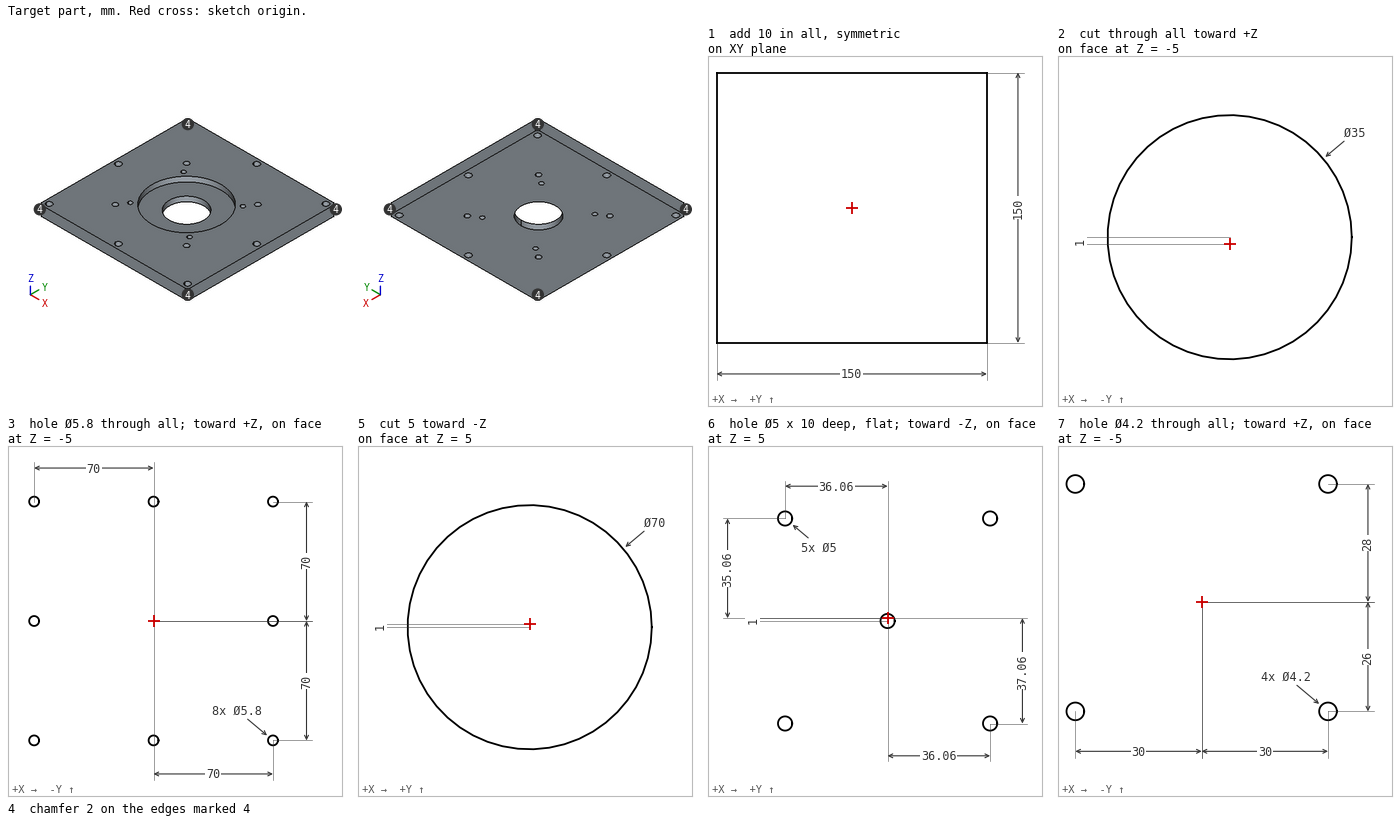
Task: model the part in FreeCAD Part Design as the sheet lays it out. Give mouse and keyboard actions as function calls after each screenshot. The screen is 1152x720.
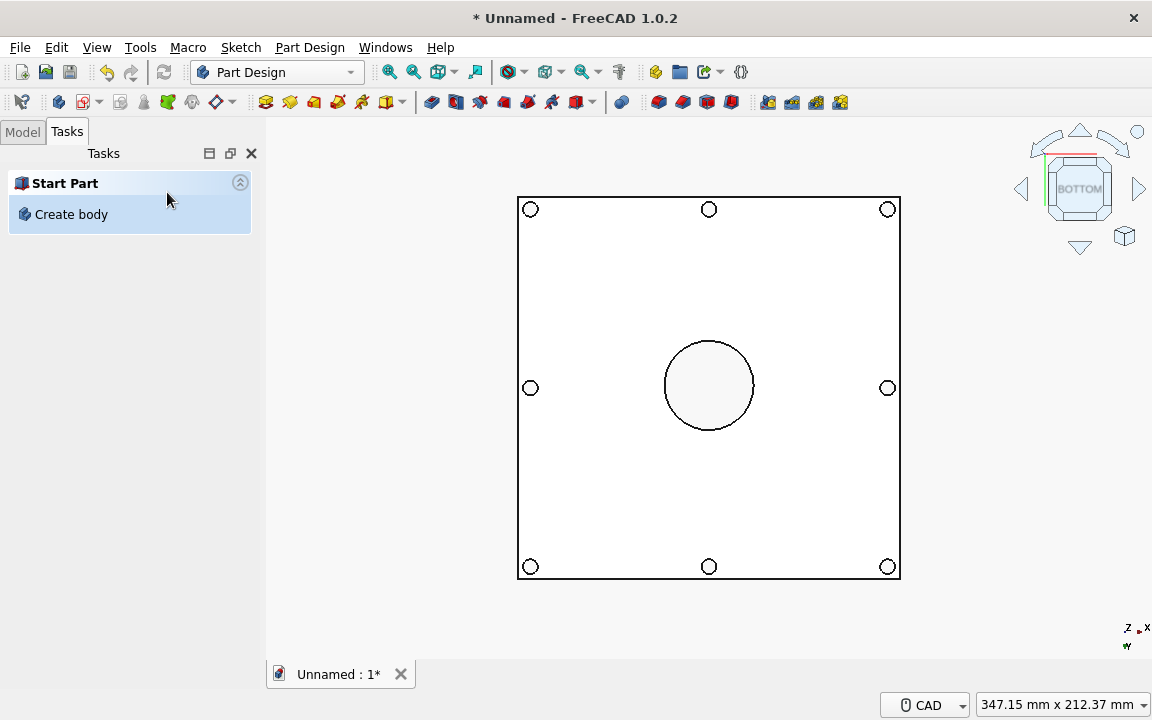
key(0)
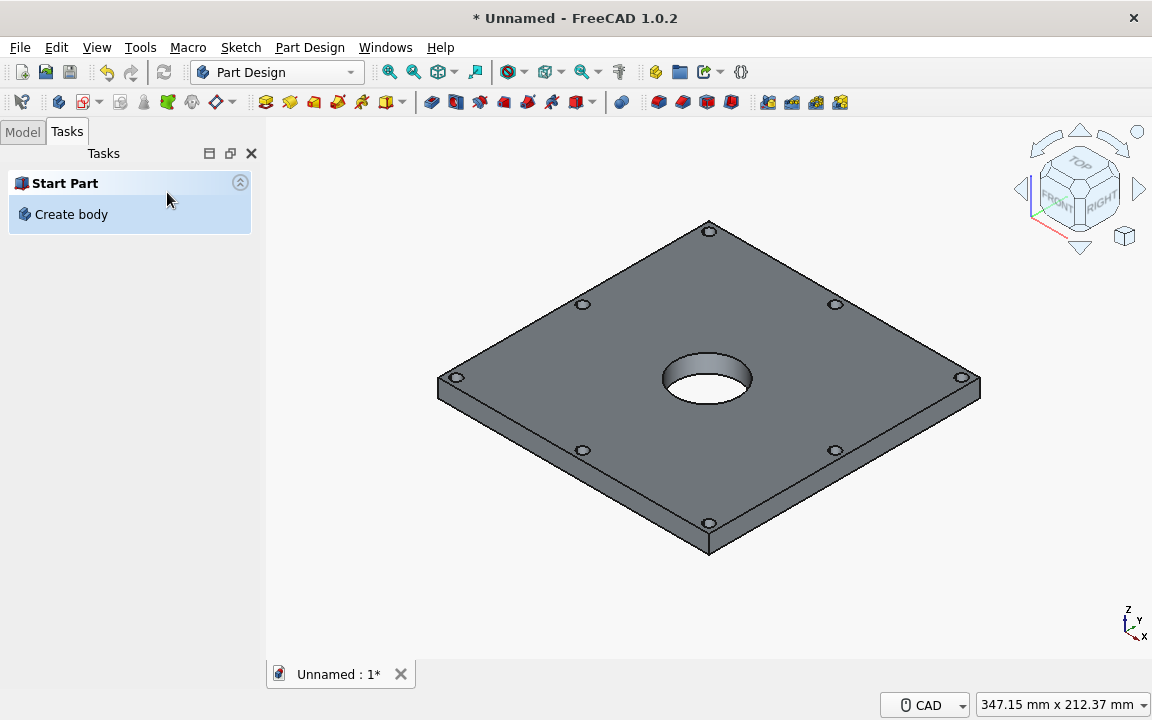
click(709, 543)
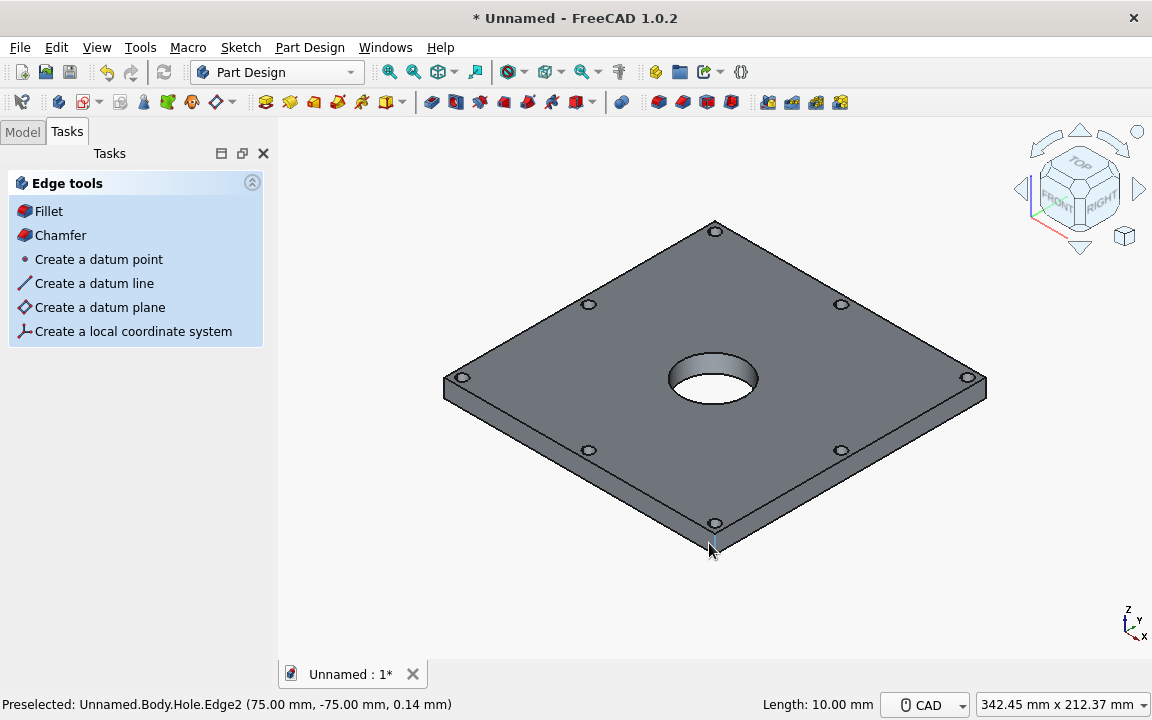
key(2)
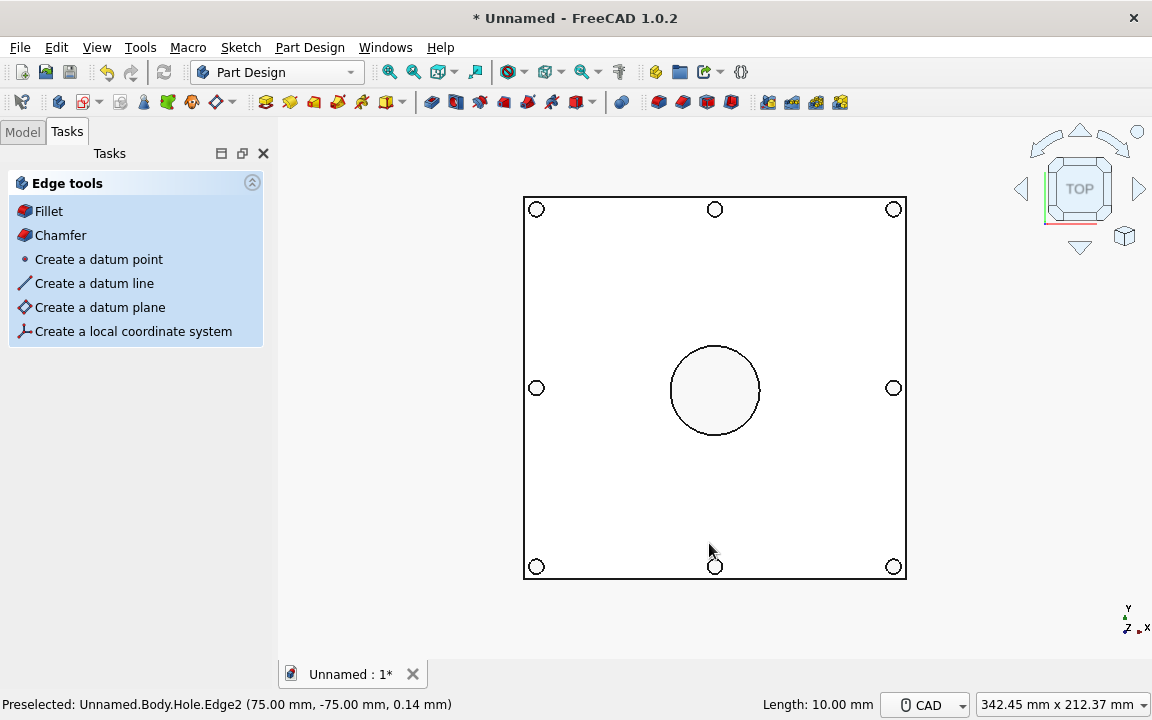
key(1)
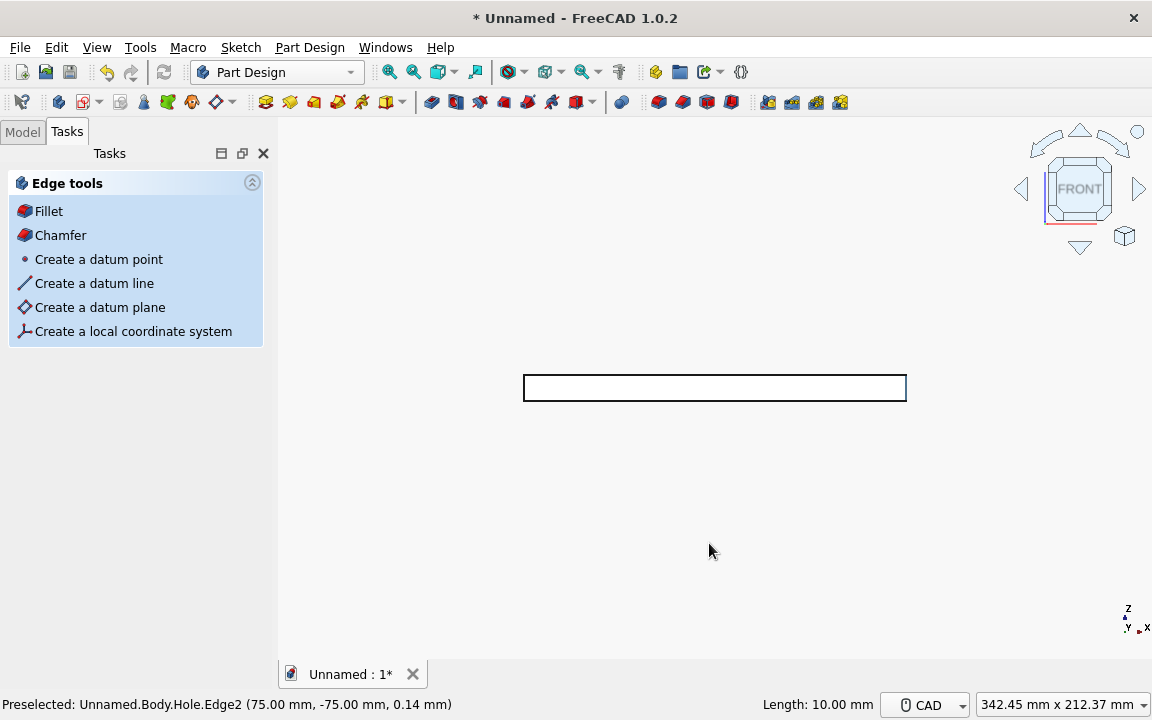
click(390, 72)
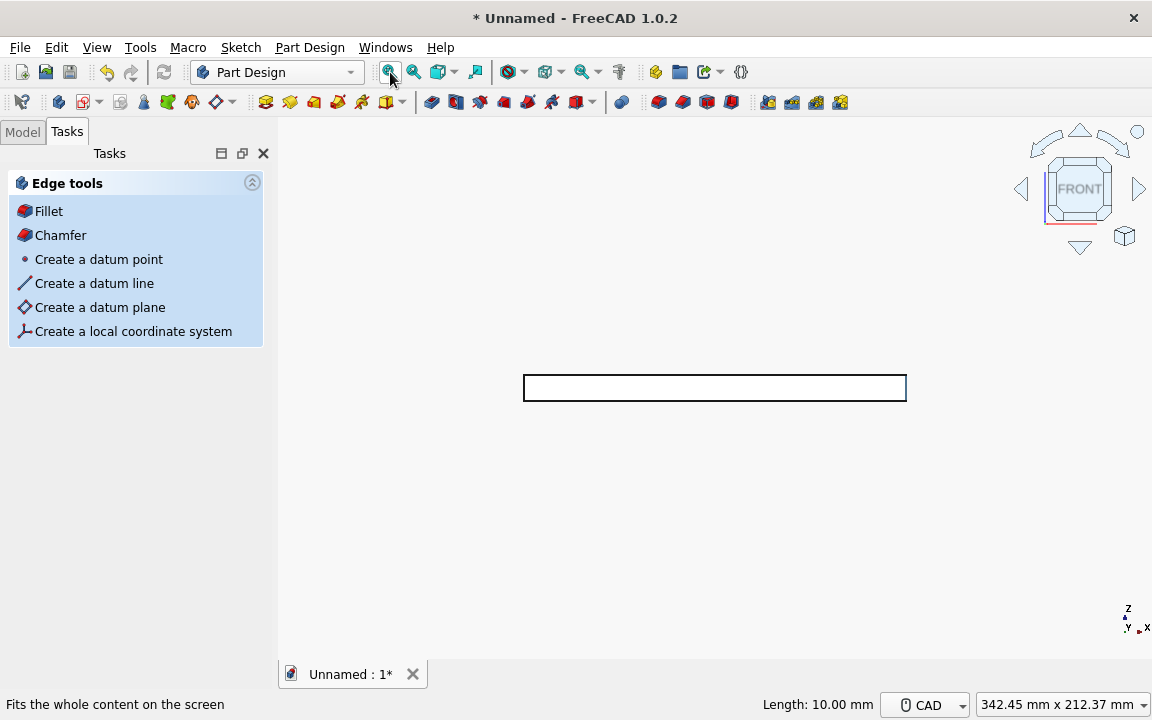
click(524, 387, ctrl)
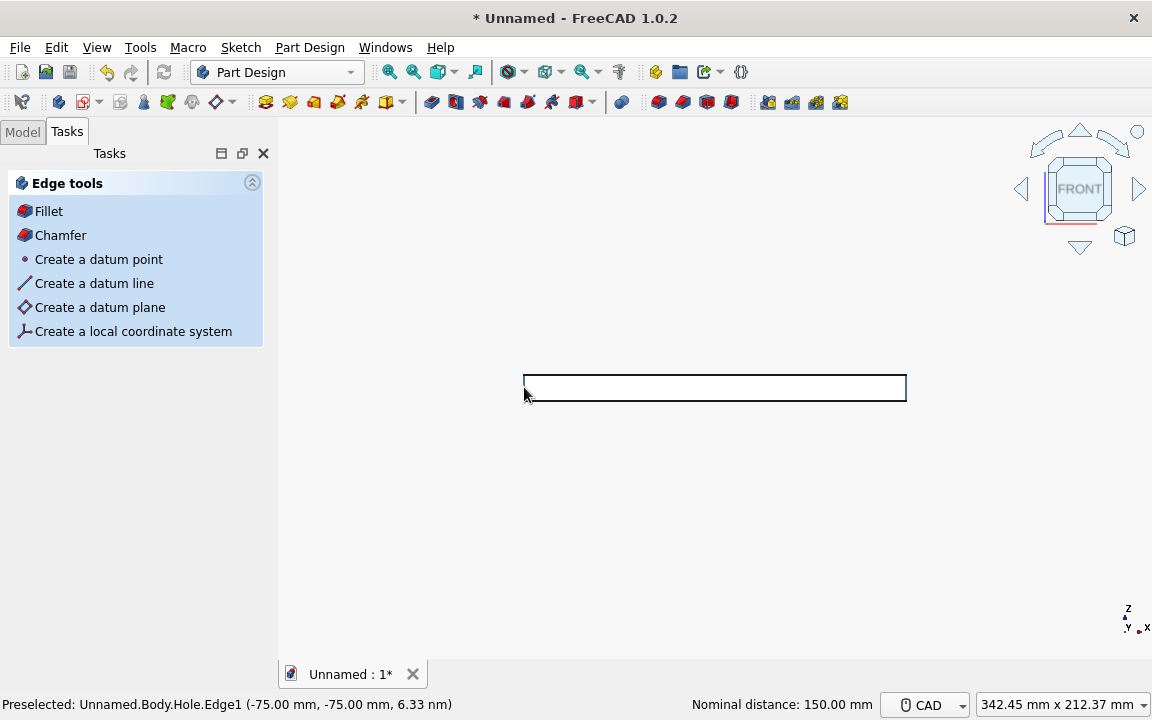
key(3)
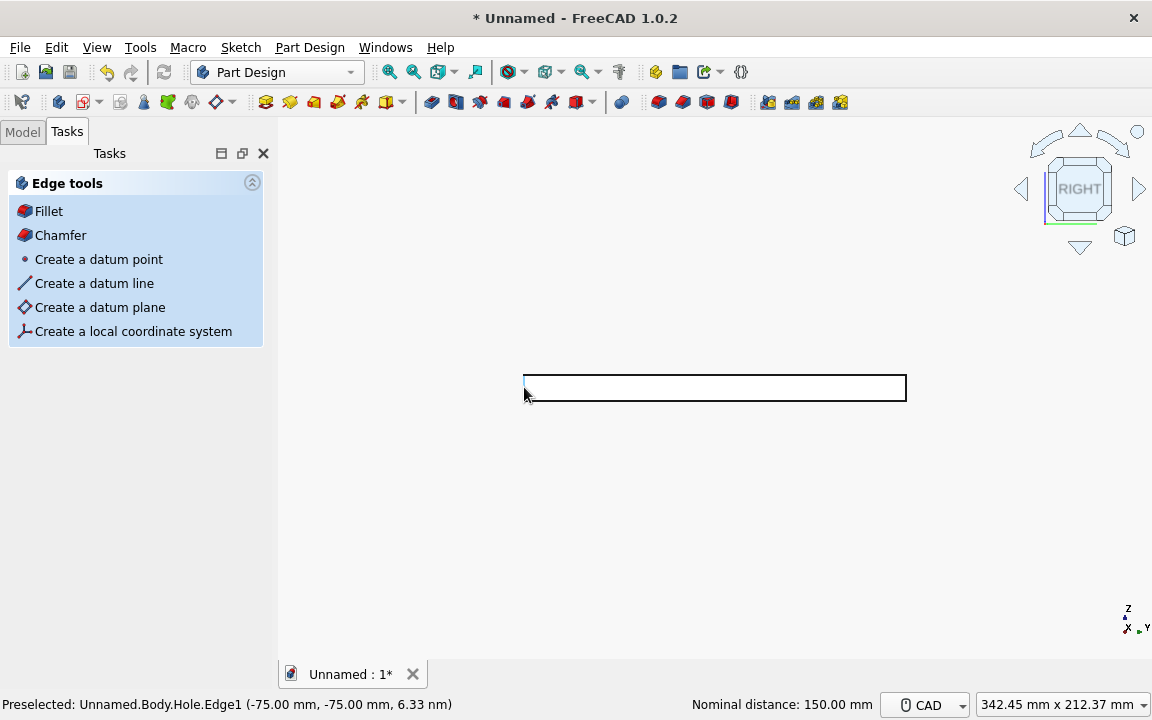
click(390, 72)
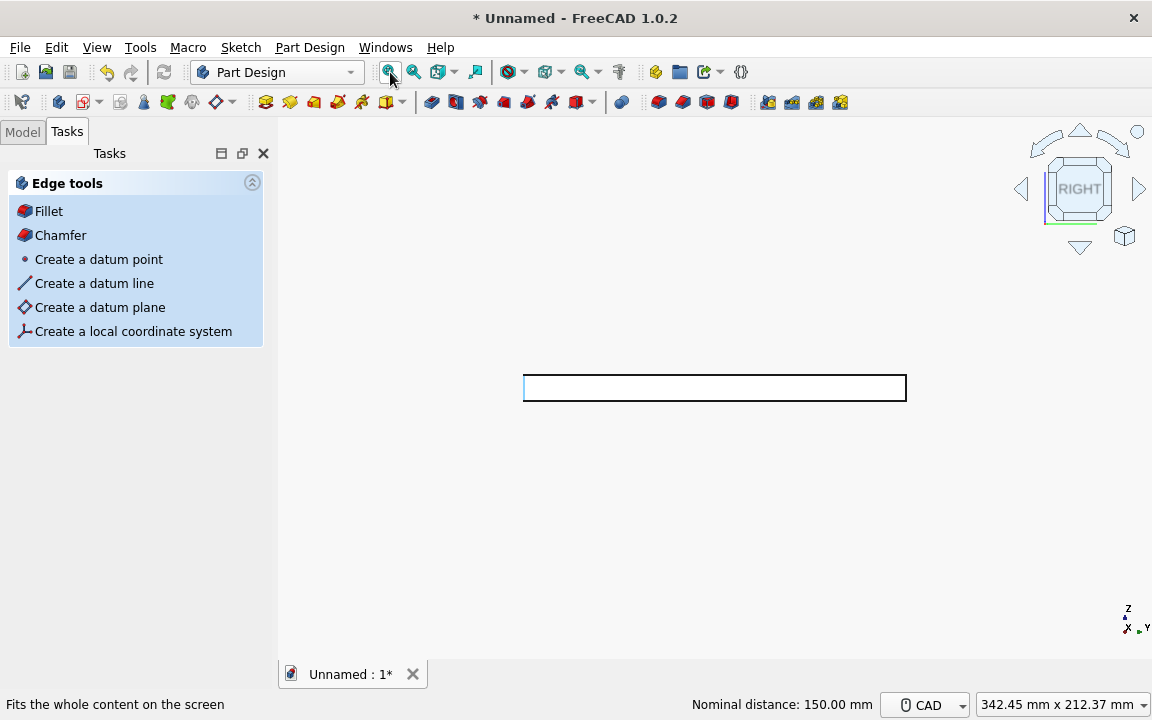
click(906, 387, ctrl)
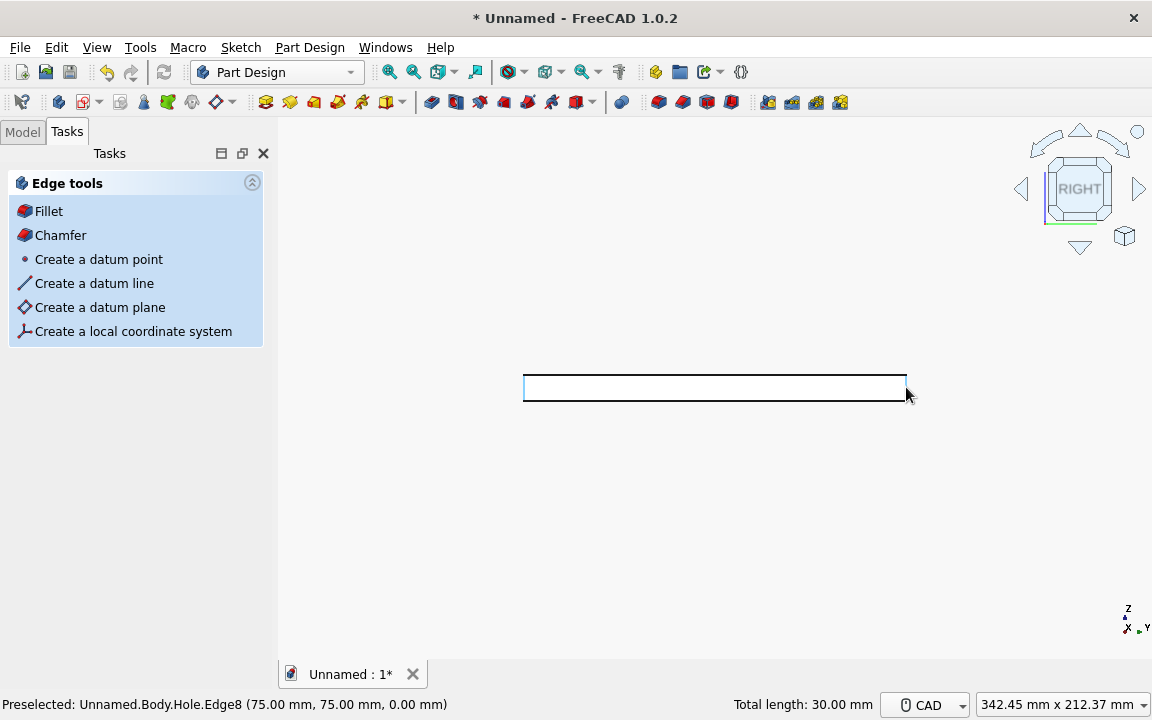
key(5)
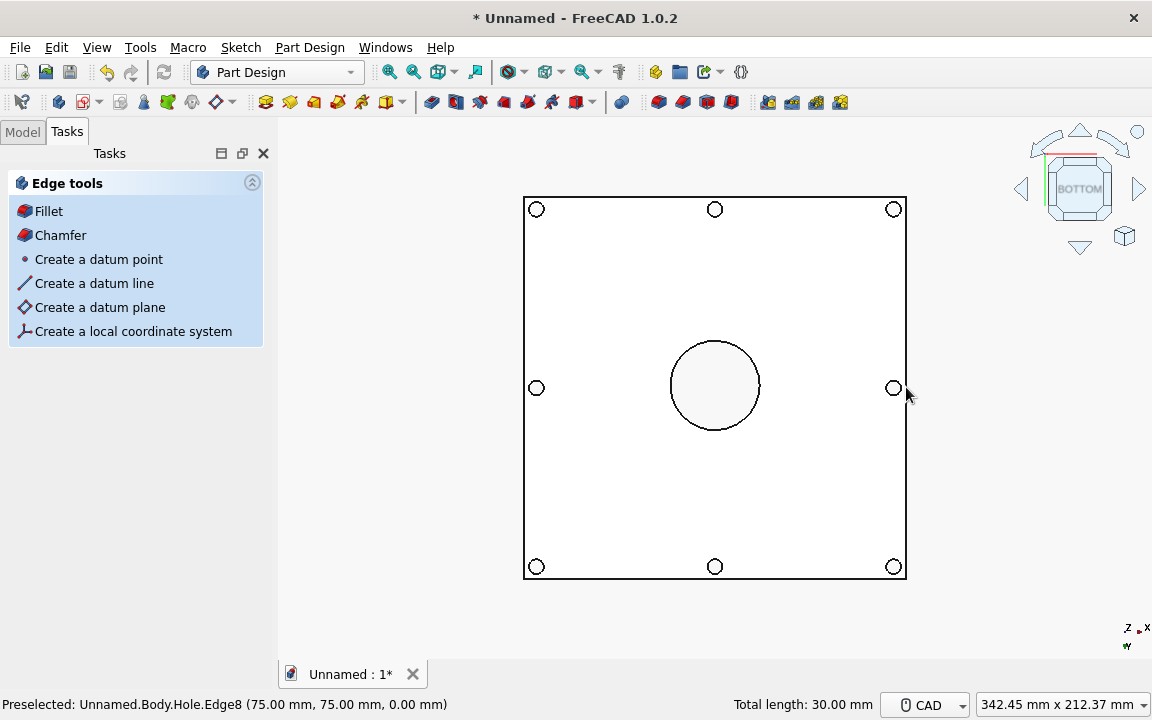
key(4)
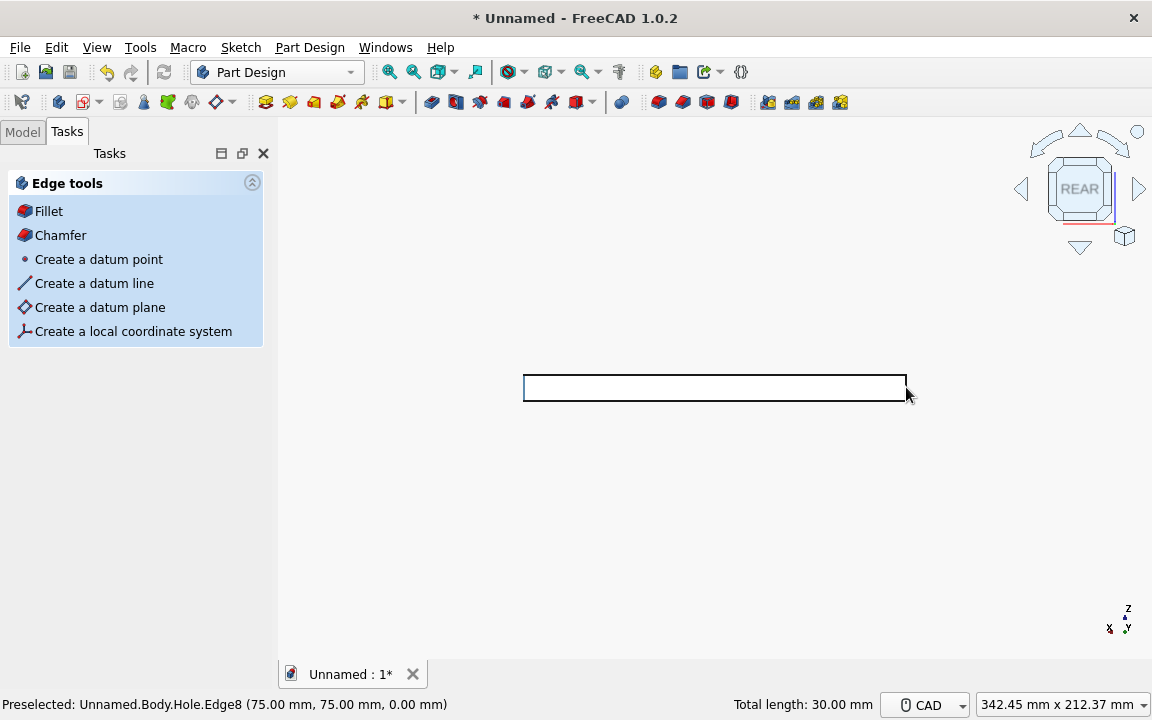
key(v)
key(f)